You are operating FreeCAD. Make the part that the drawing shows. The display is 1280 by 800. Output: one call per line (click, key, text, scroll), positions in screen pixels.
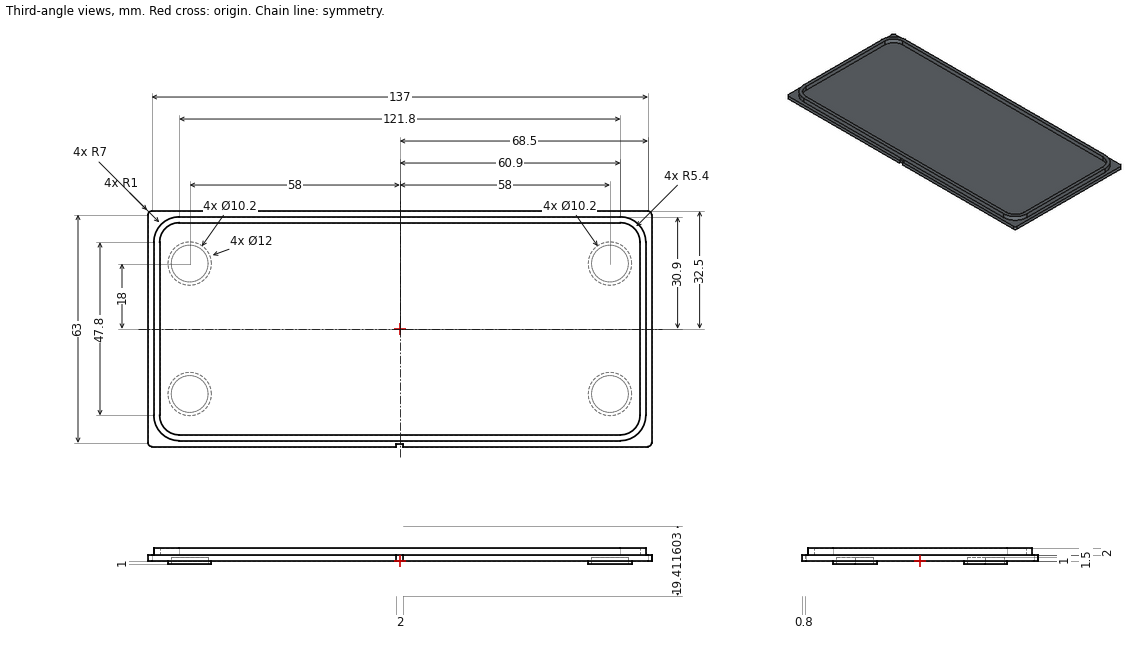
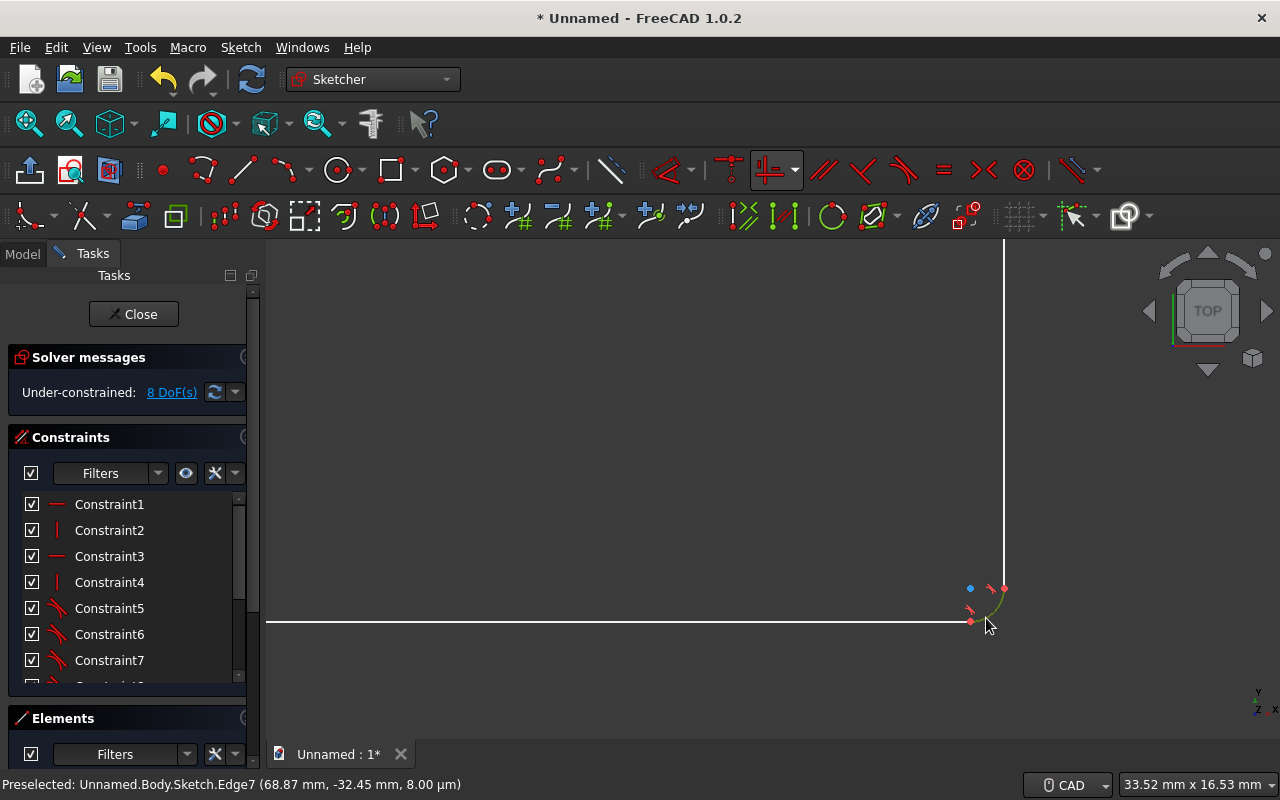
scroll(987, 622, down, 10)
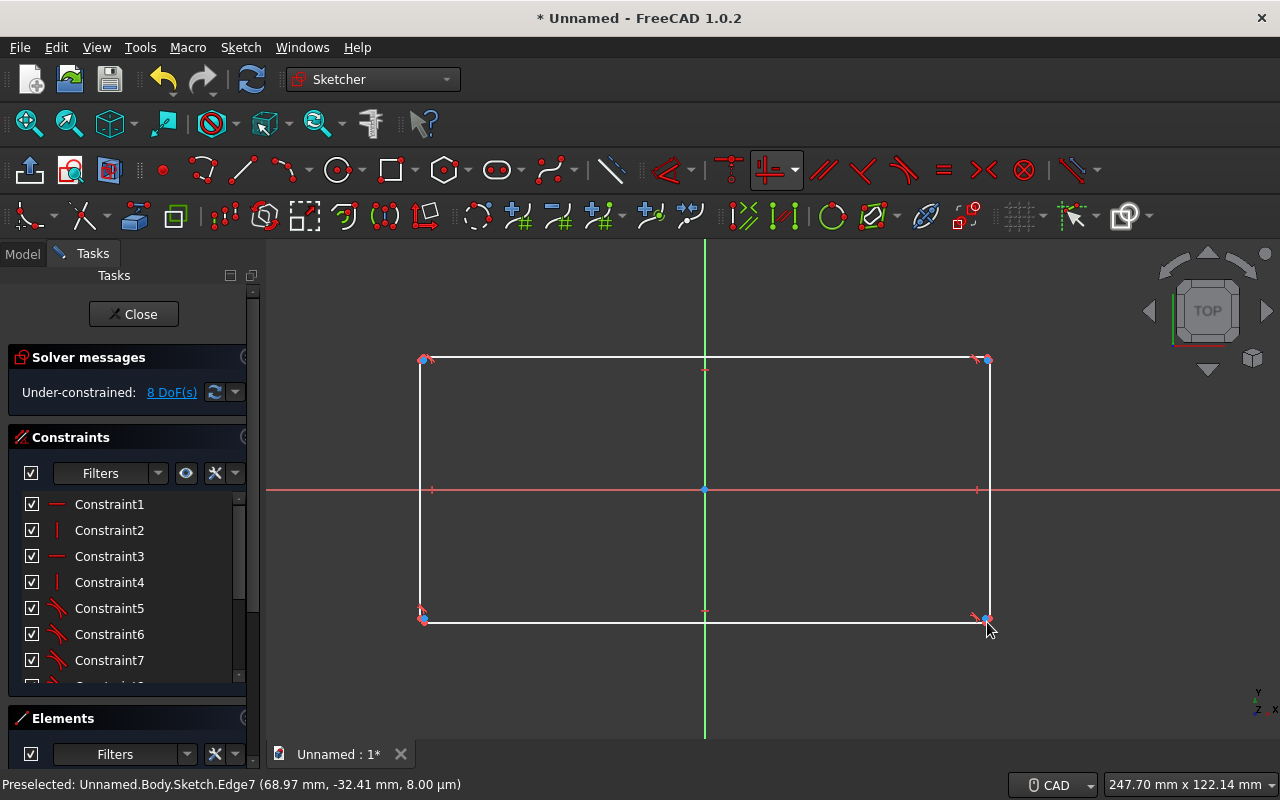
scroll(990, 359, up, 12)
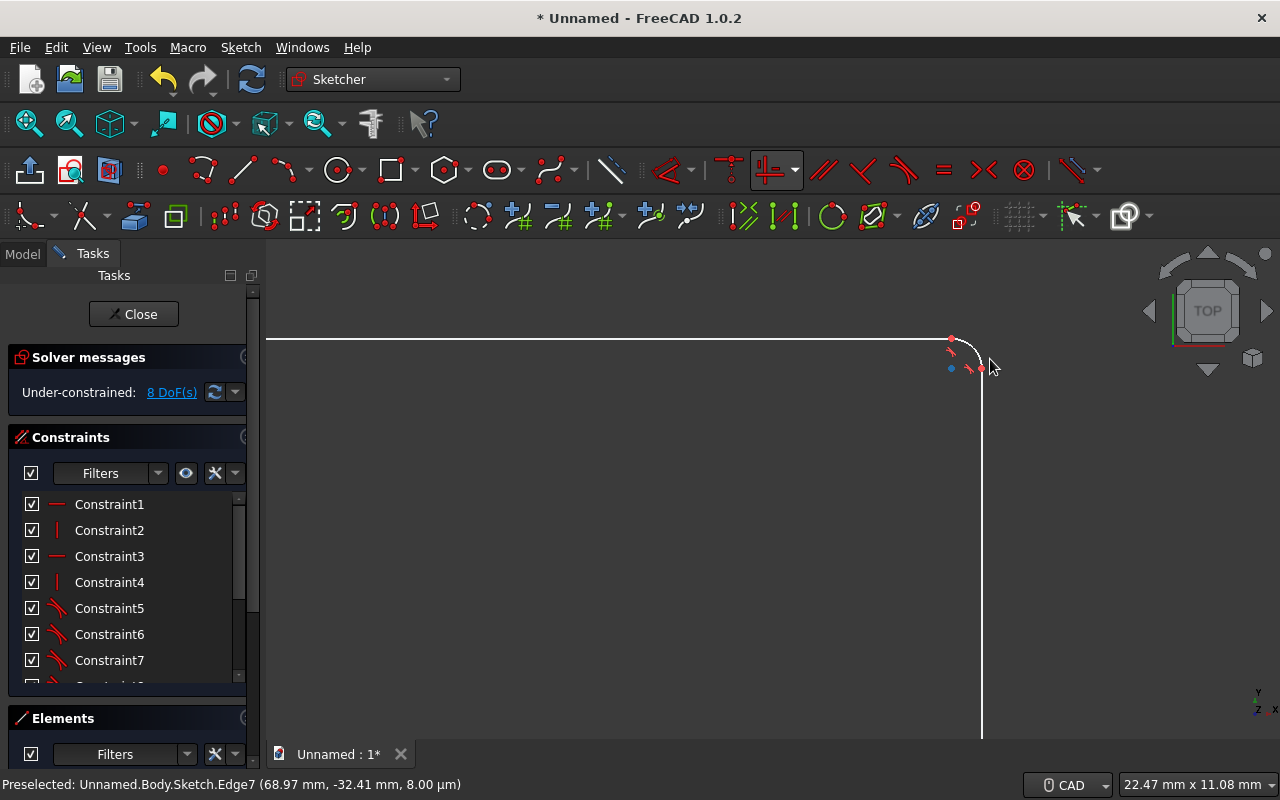
click(979, 355)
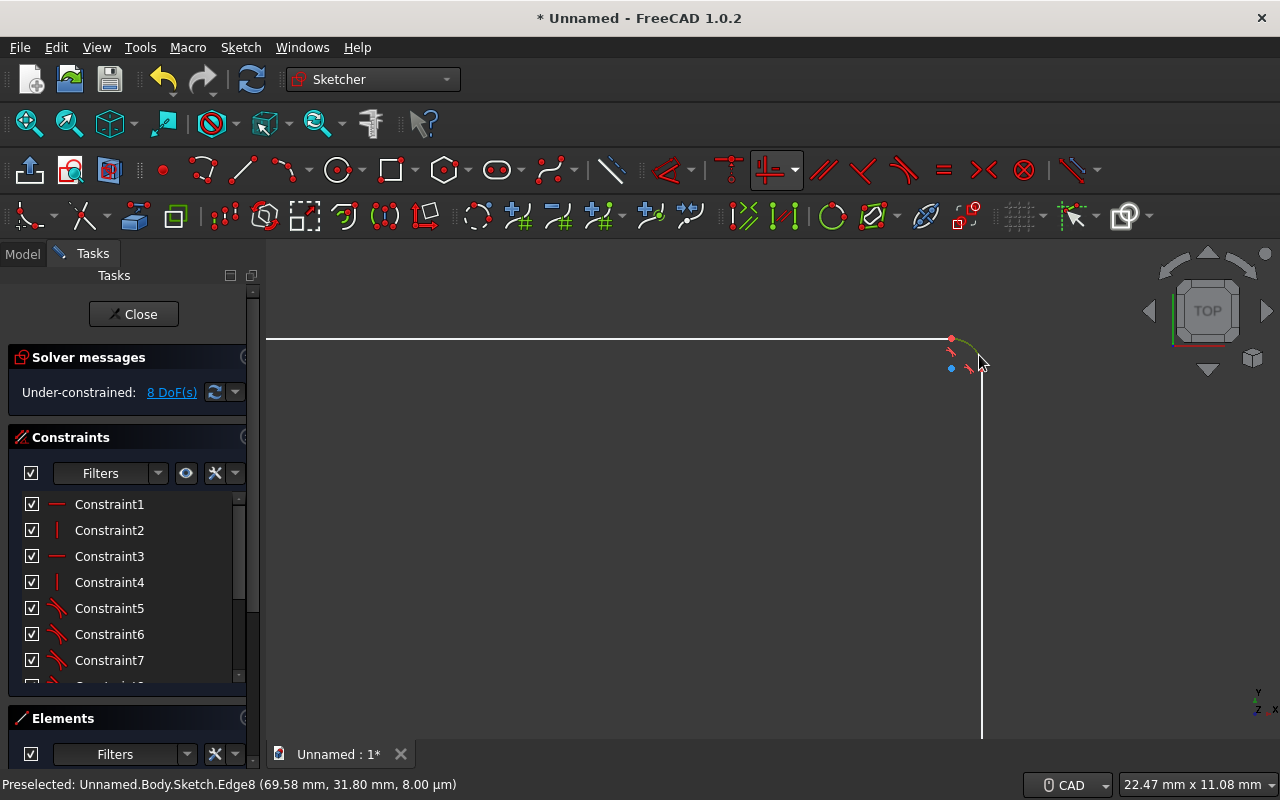
click(944, 170)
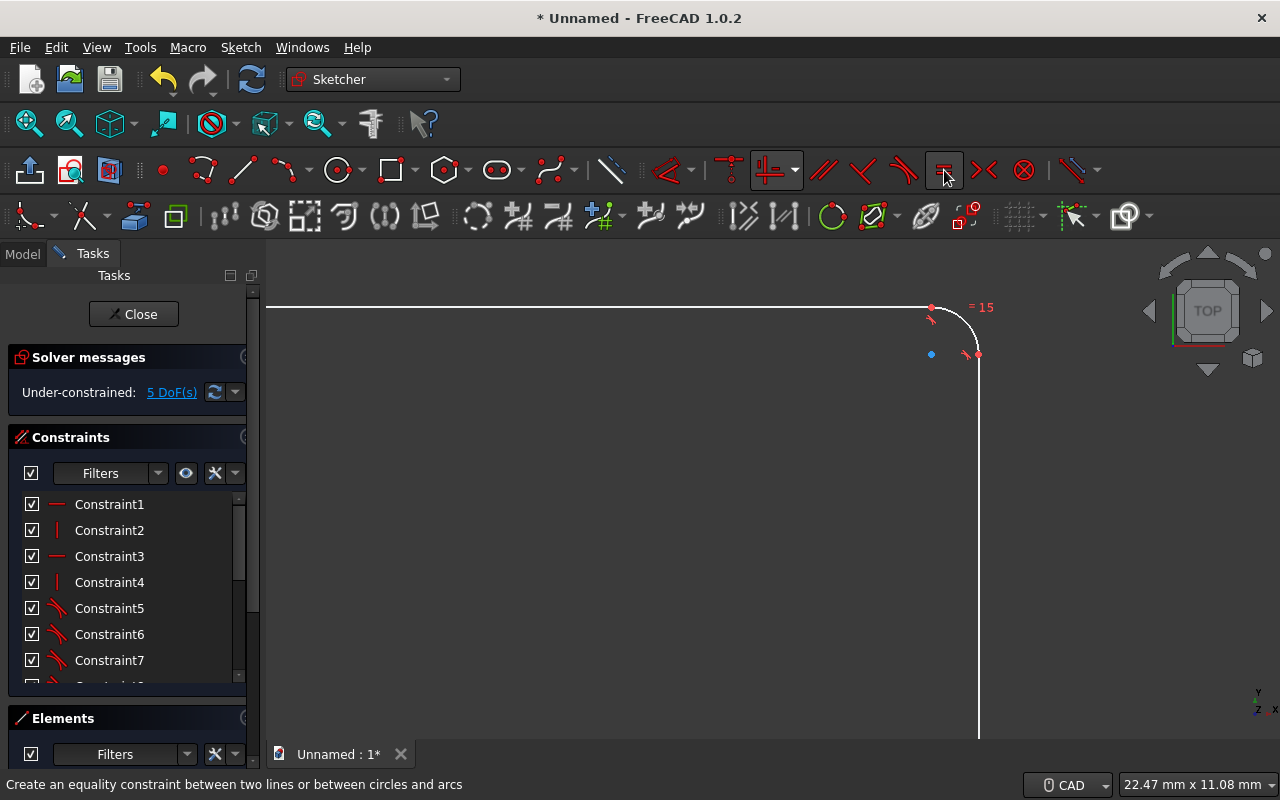
click(666, 170)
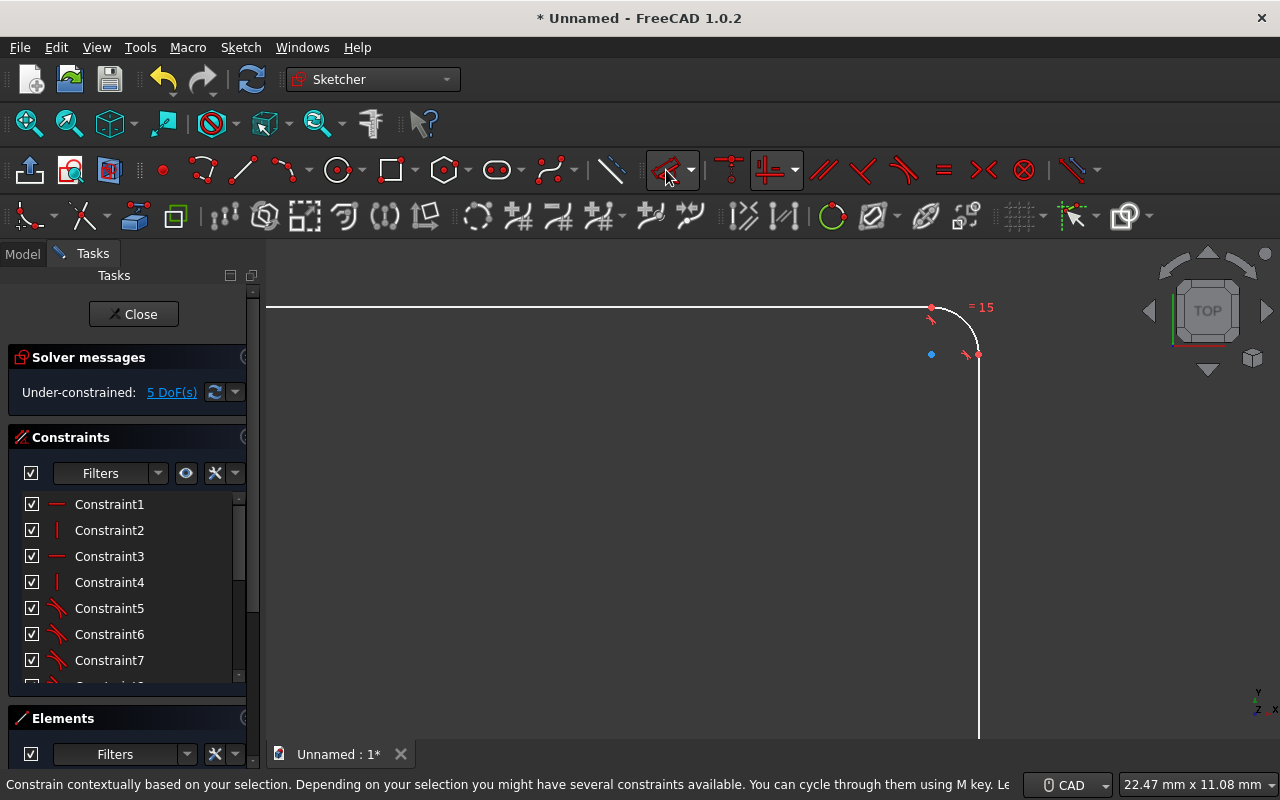
scroll(990, 359, down, 12)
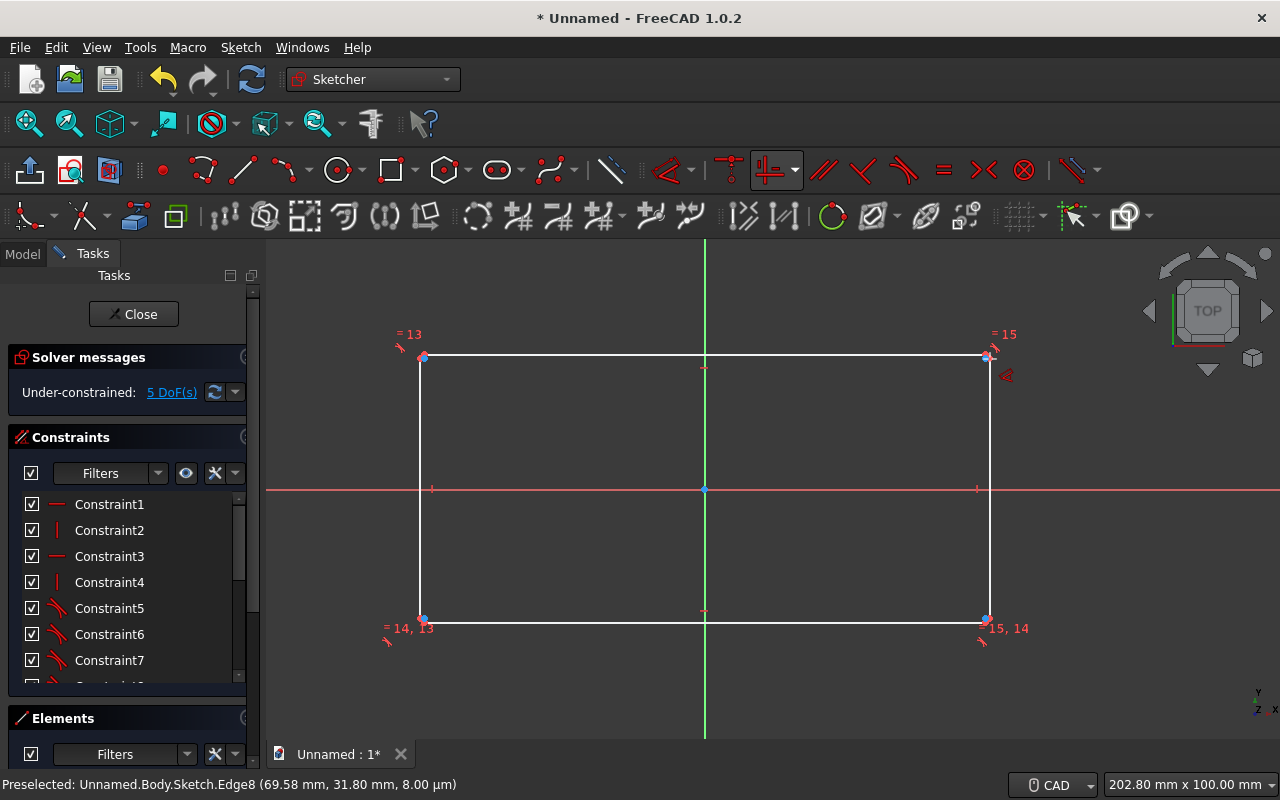
scroll(423, 355, up, 12)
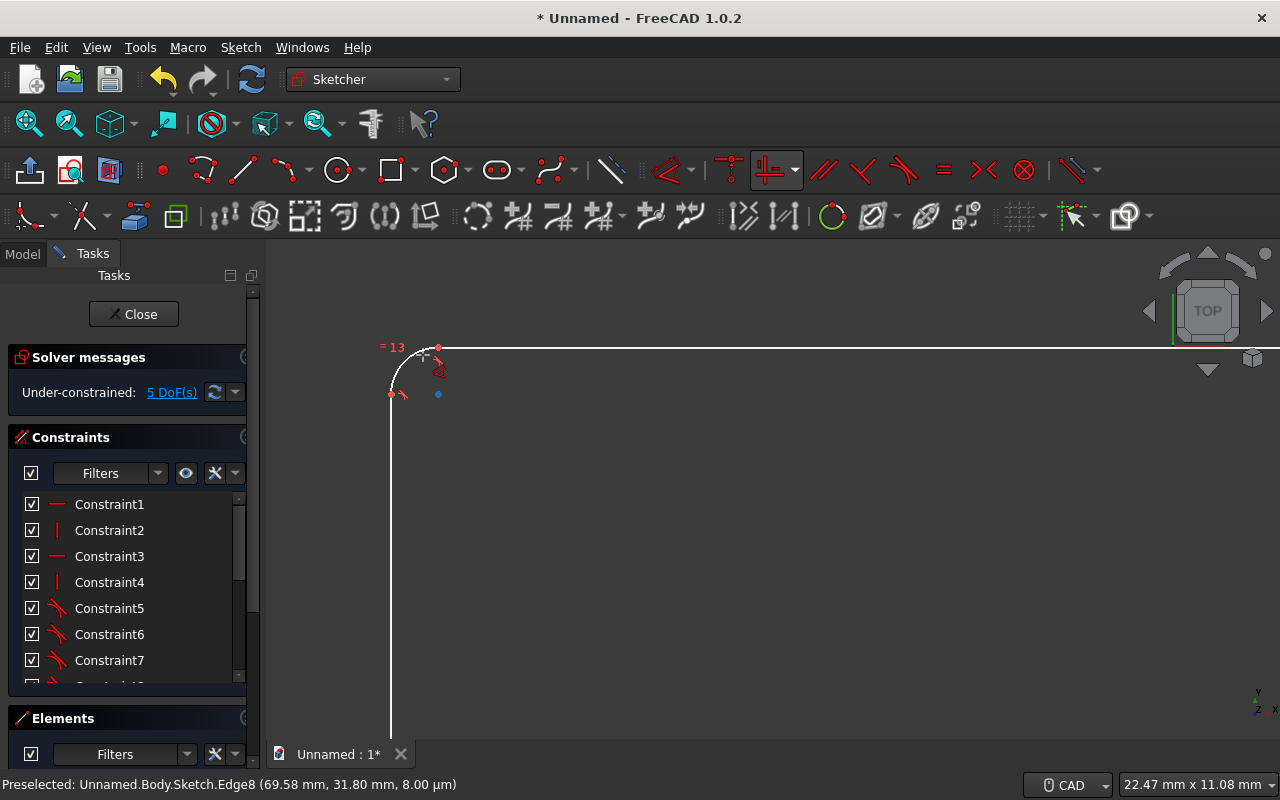
click(417, 353)
click(403, 324)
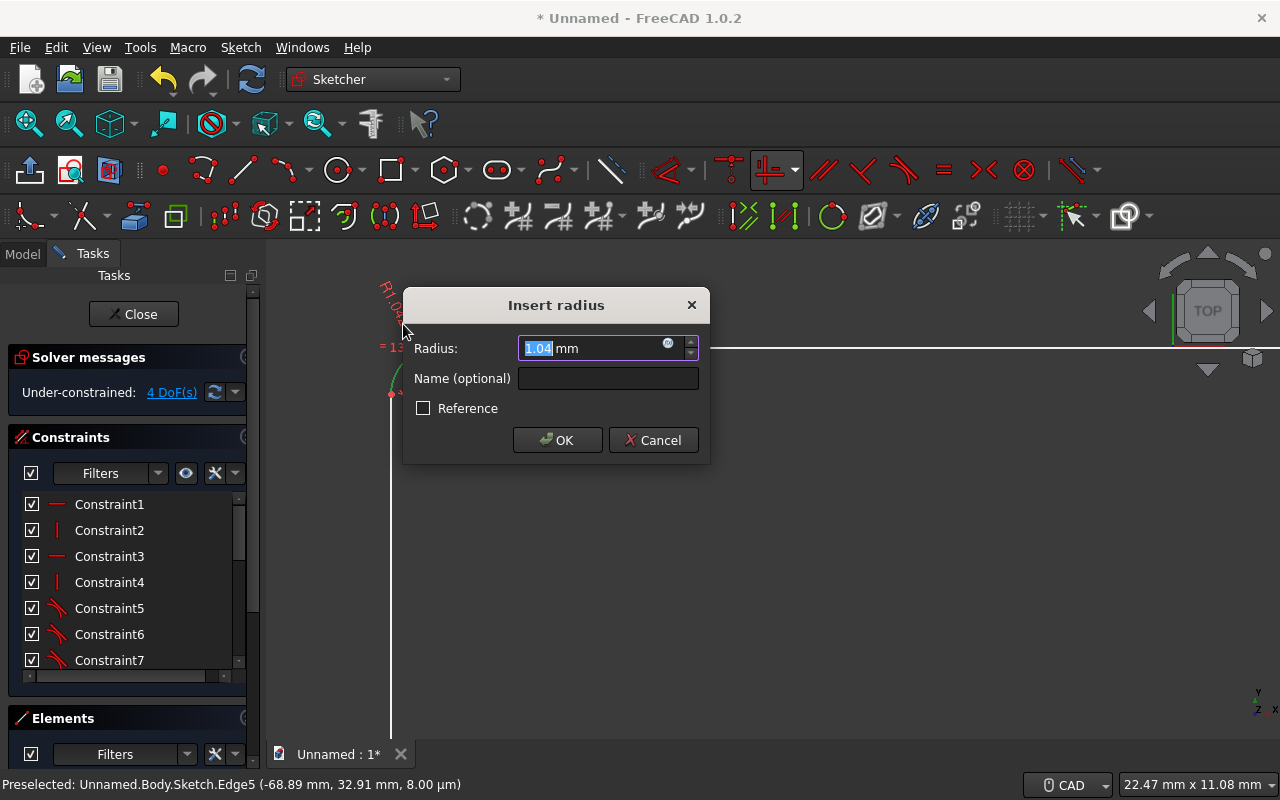
text(1)
key(Return)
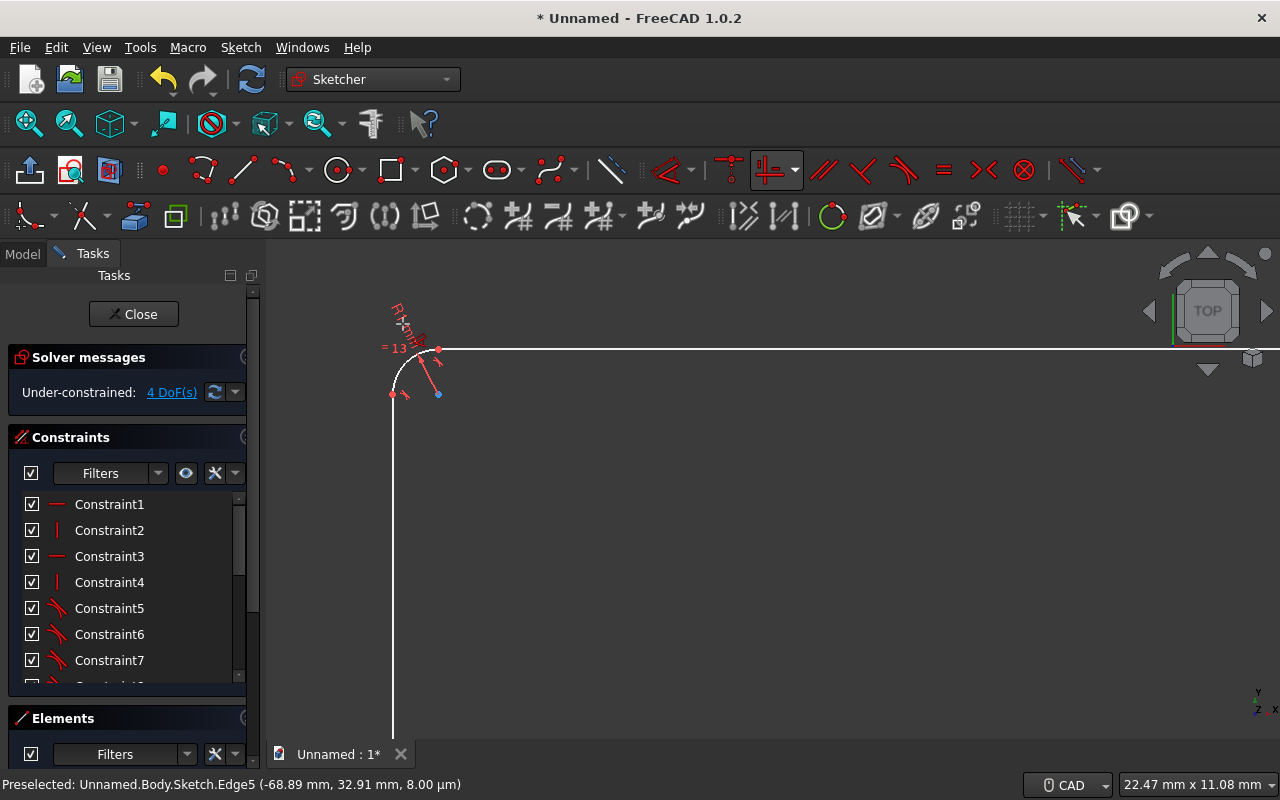
scroll(423, 355, down, 12)